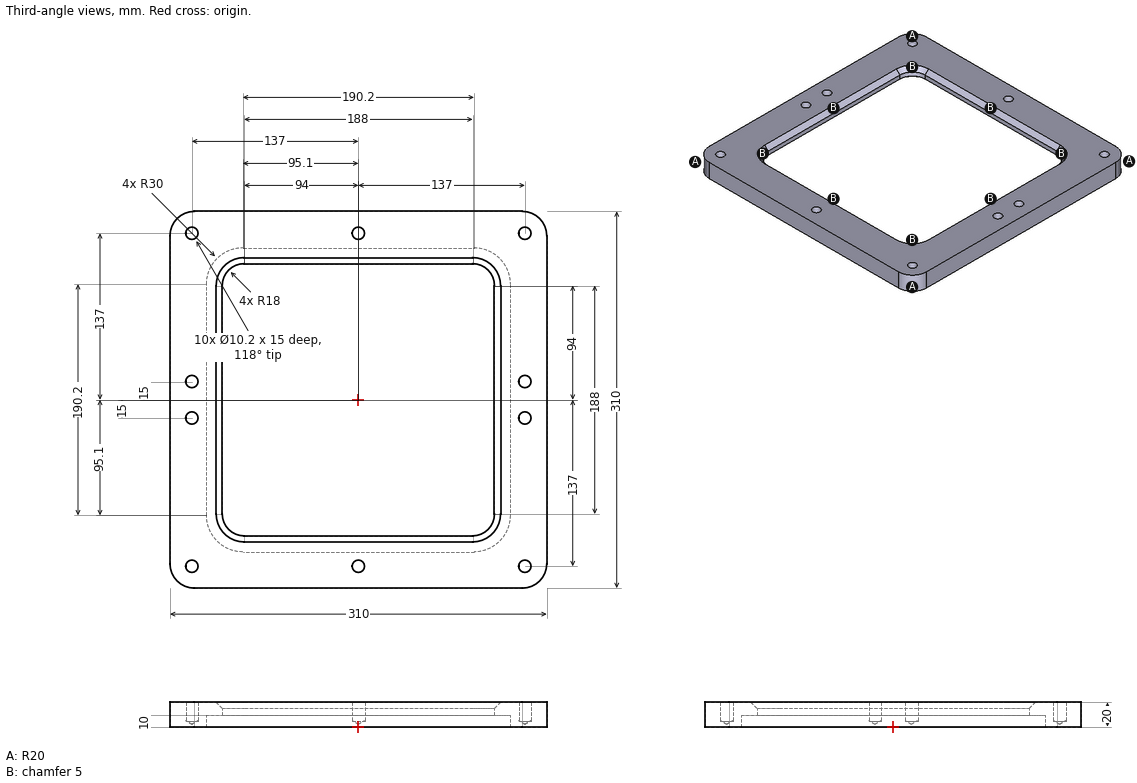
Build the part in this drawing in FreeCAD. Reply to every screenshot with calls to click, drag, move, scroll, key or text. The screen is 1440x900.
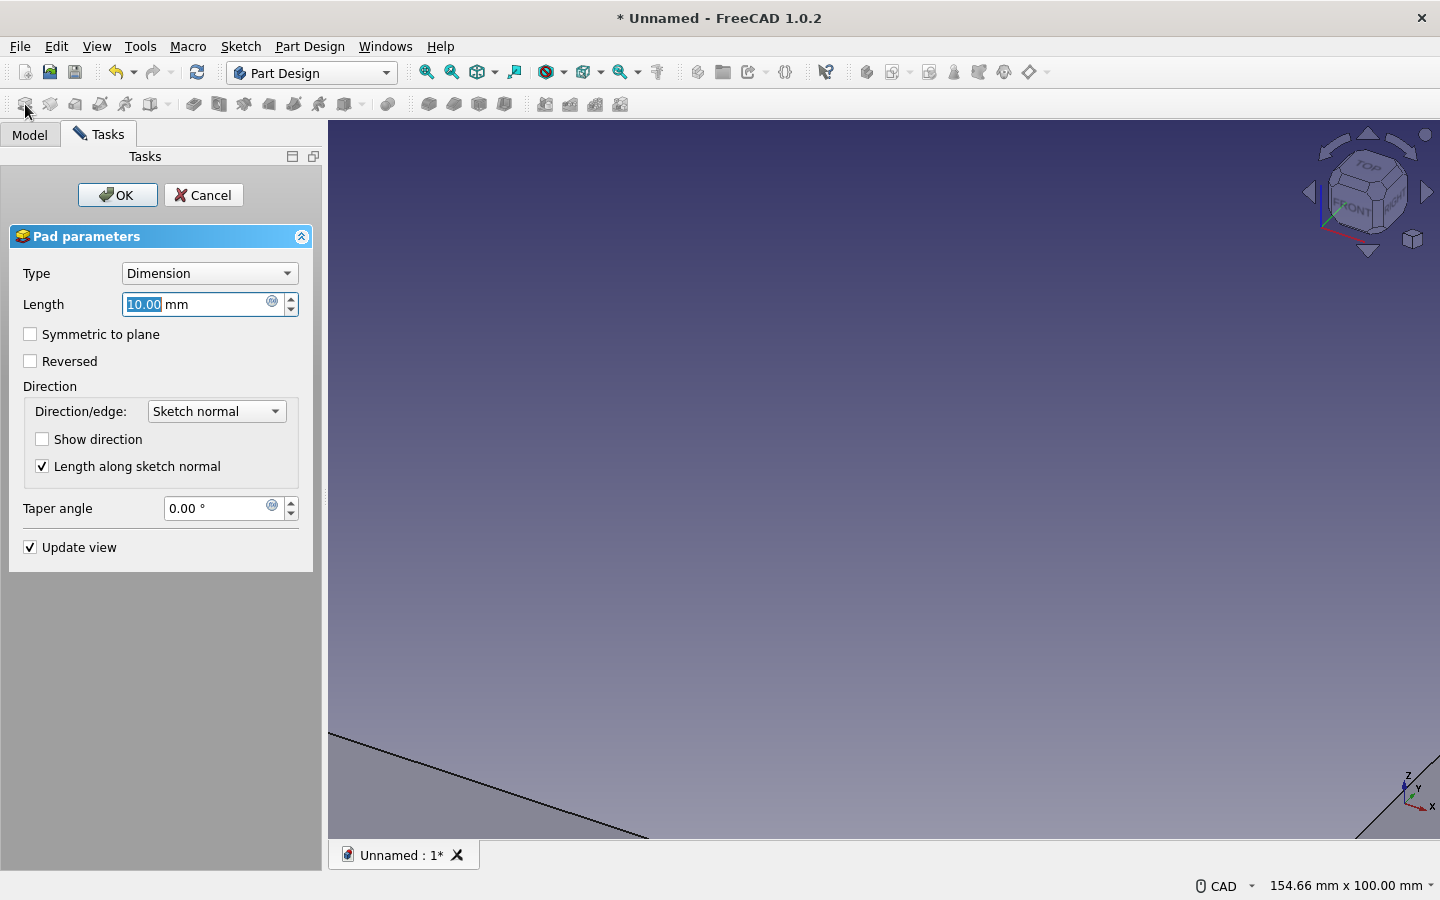
text(20)
key(Tab)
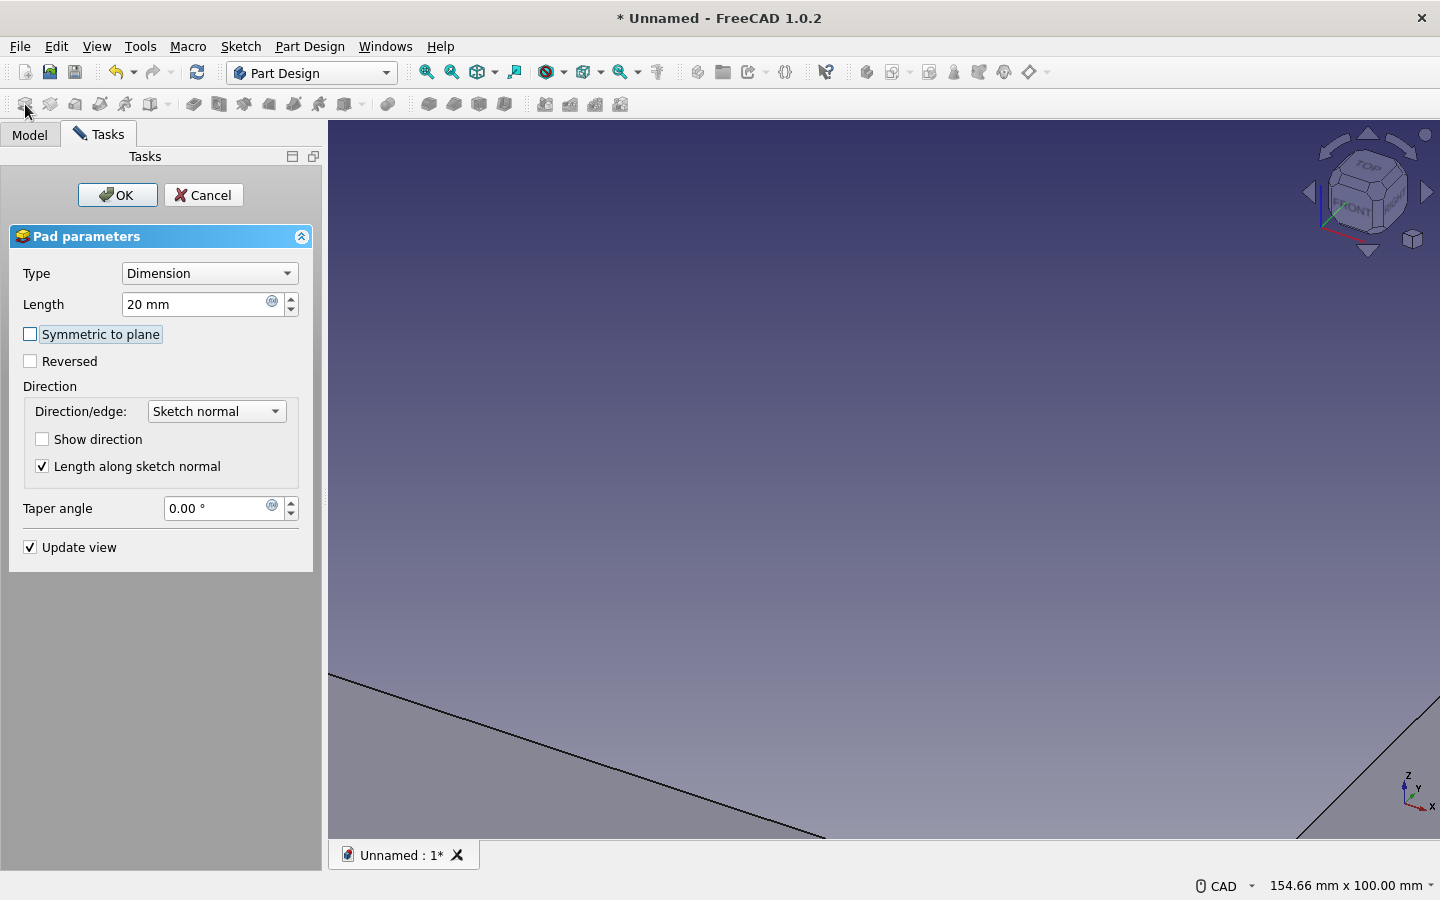
click(118, 195)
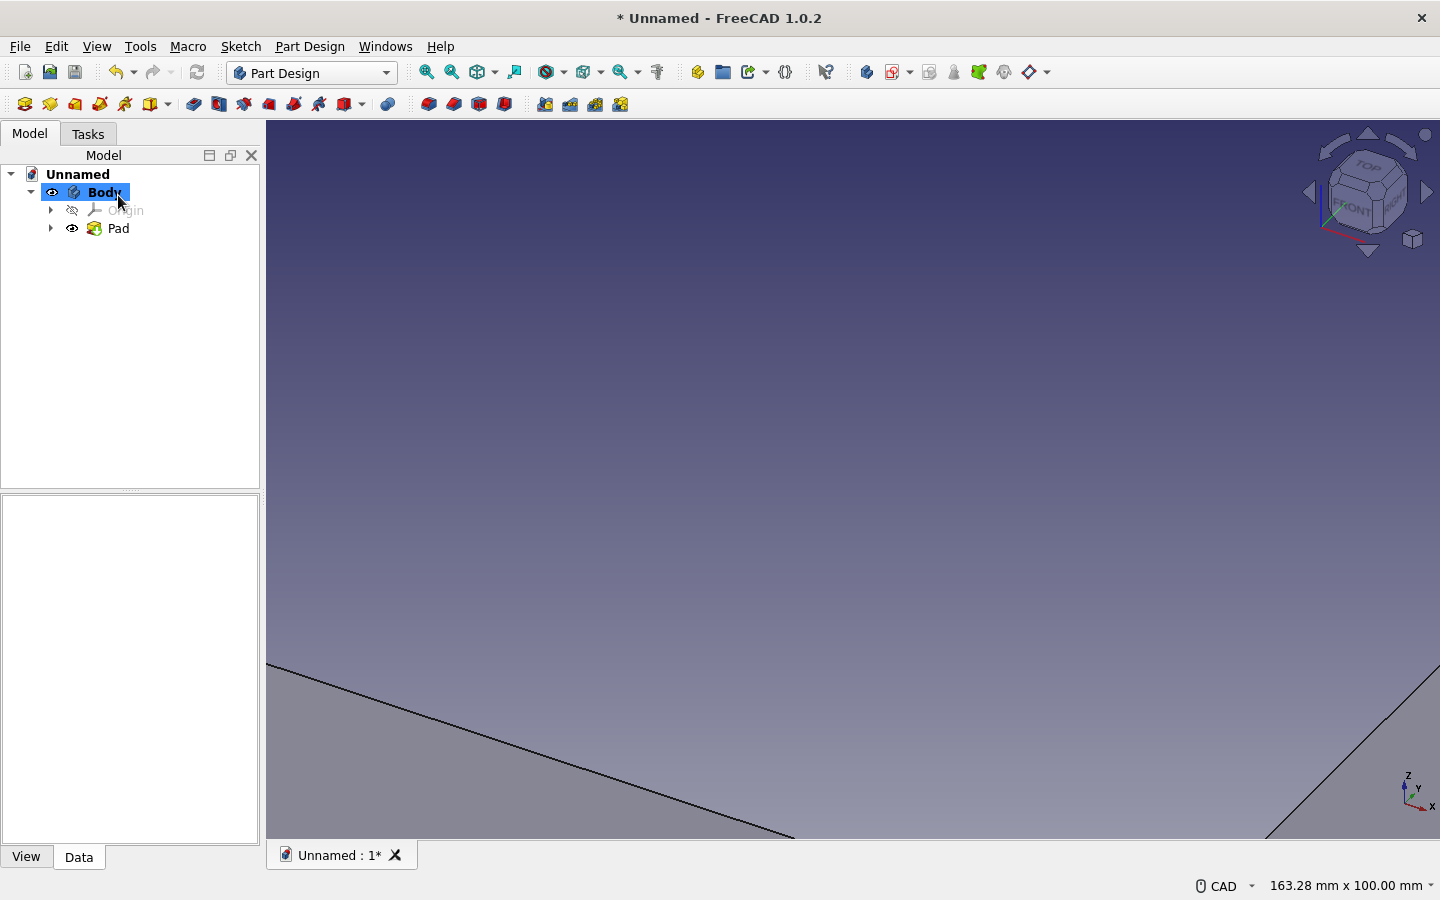
click(427, 72)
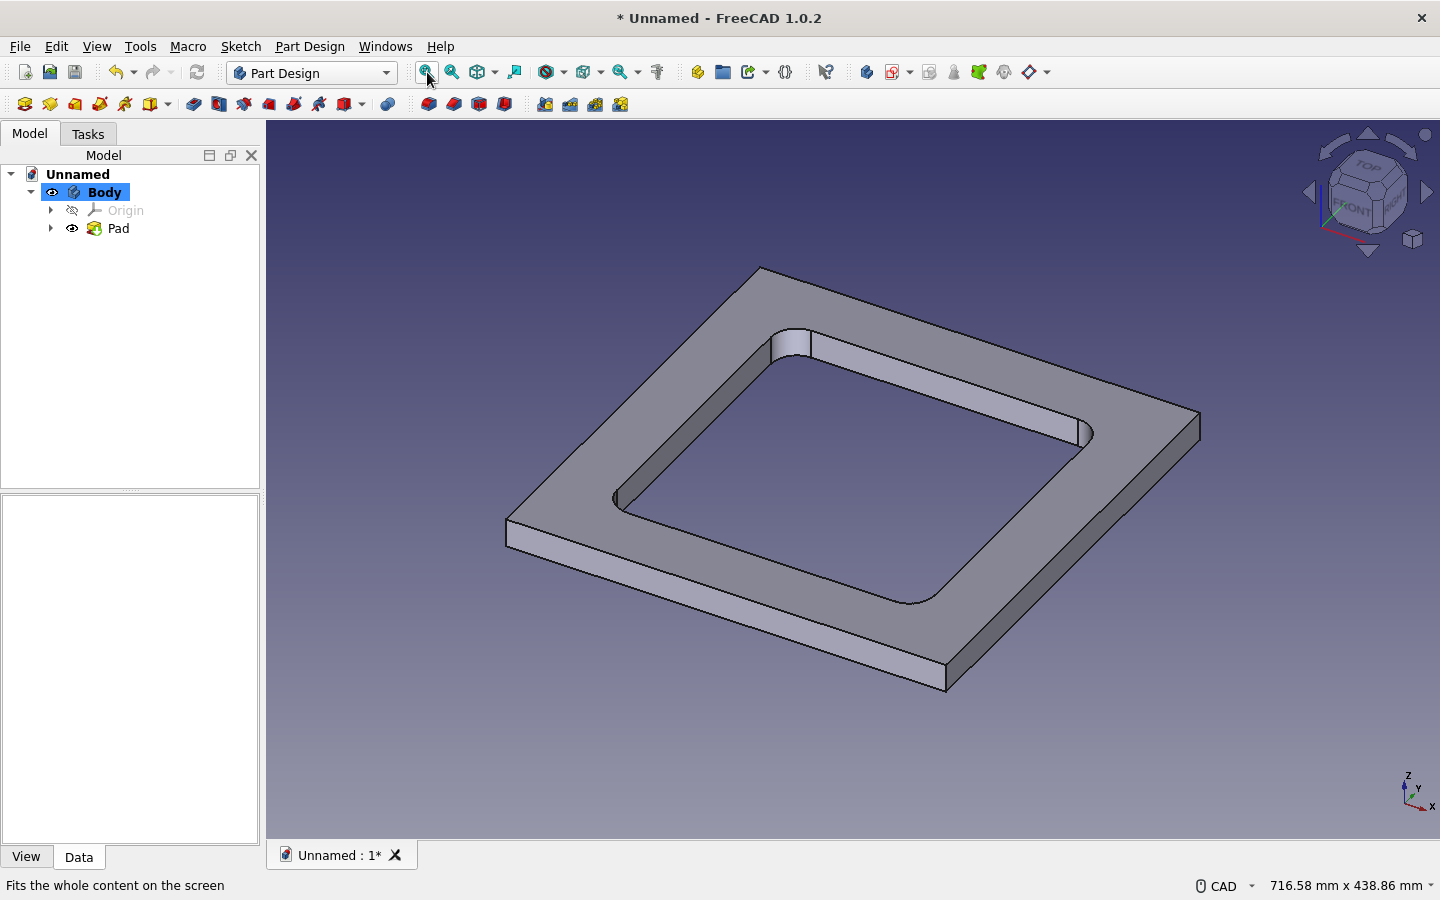
click(946, 677)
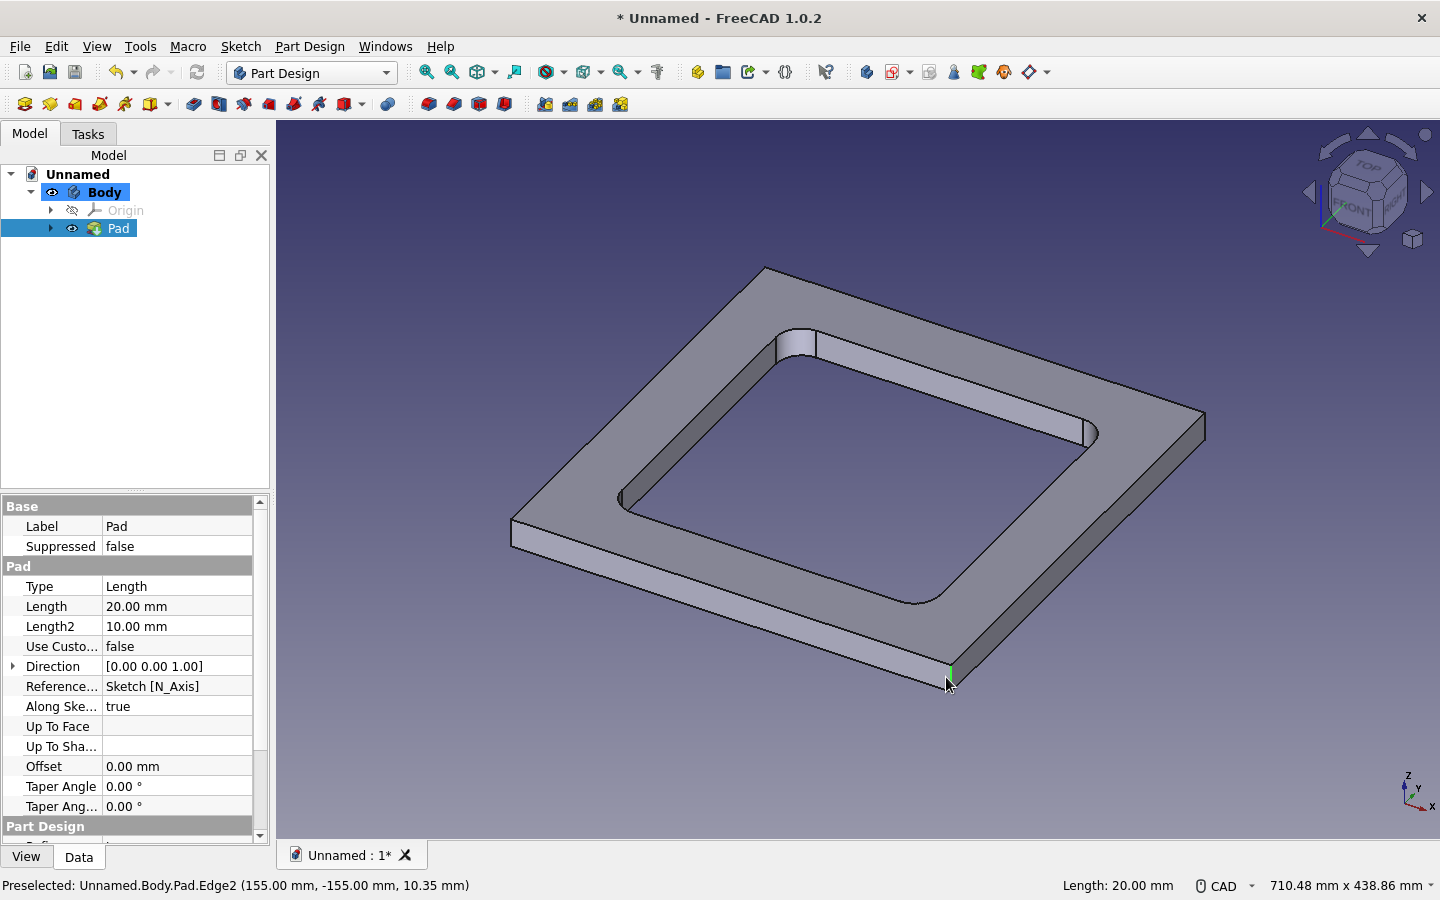
key(0)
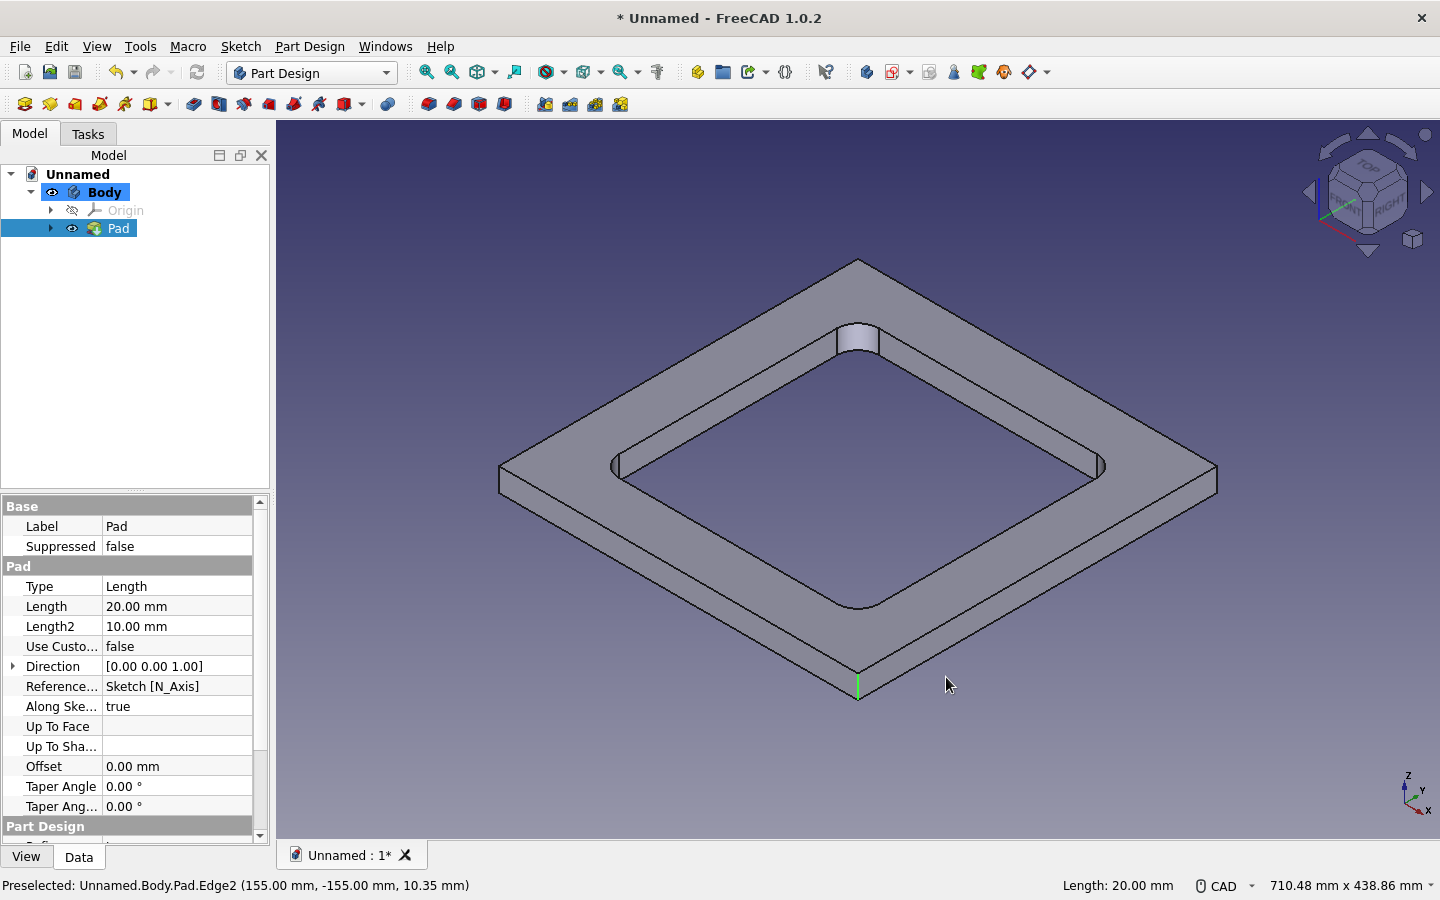
key(2)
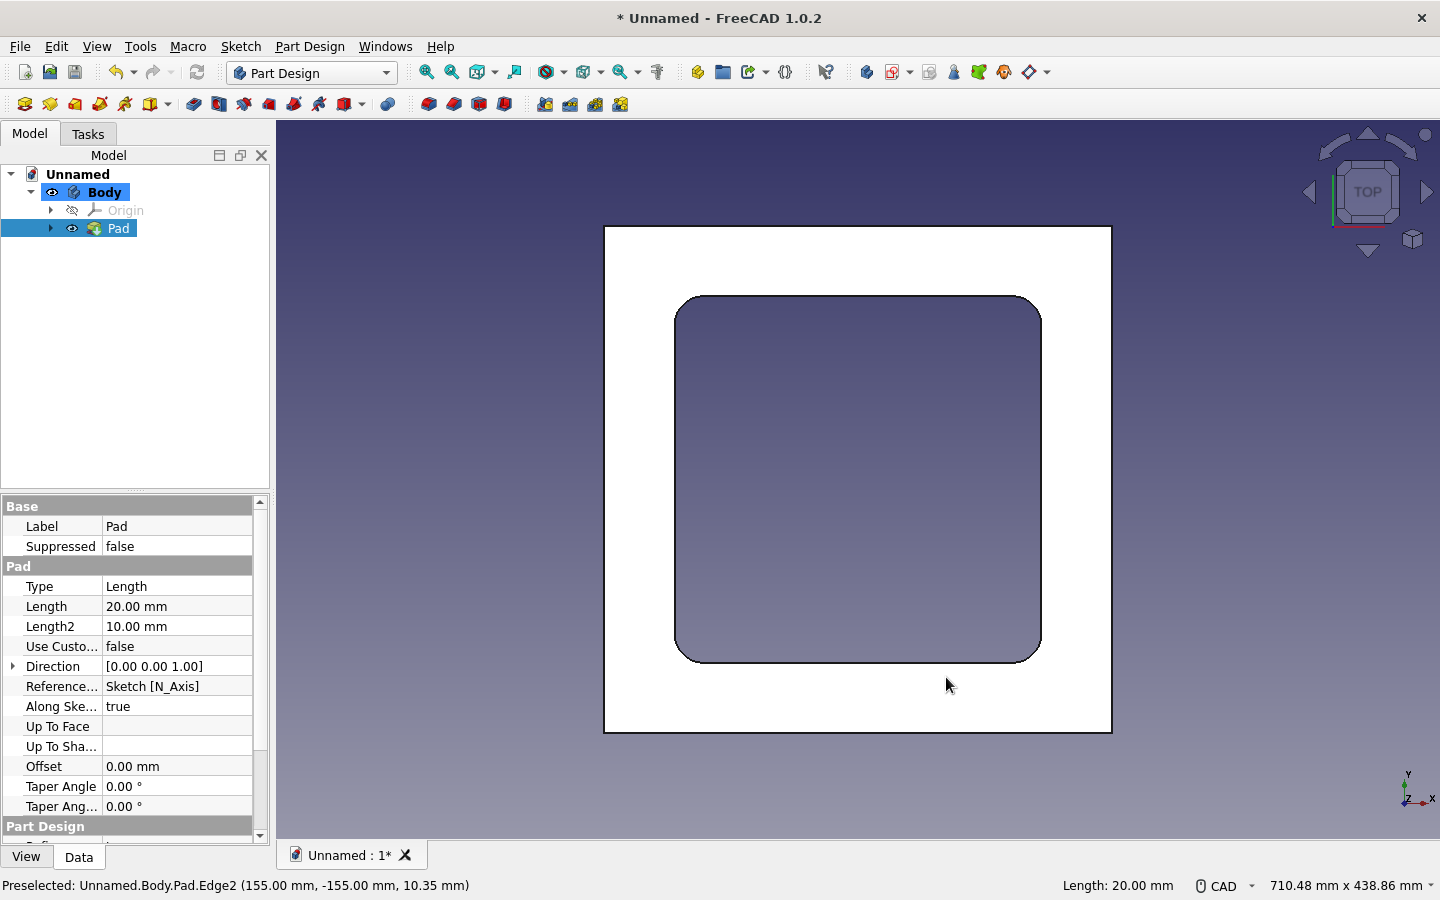
key(1)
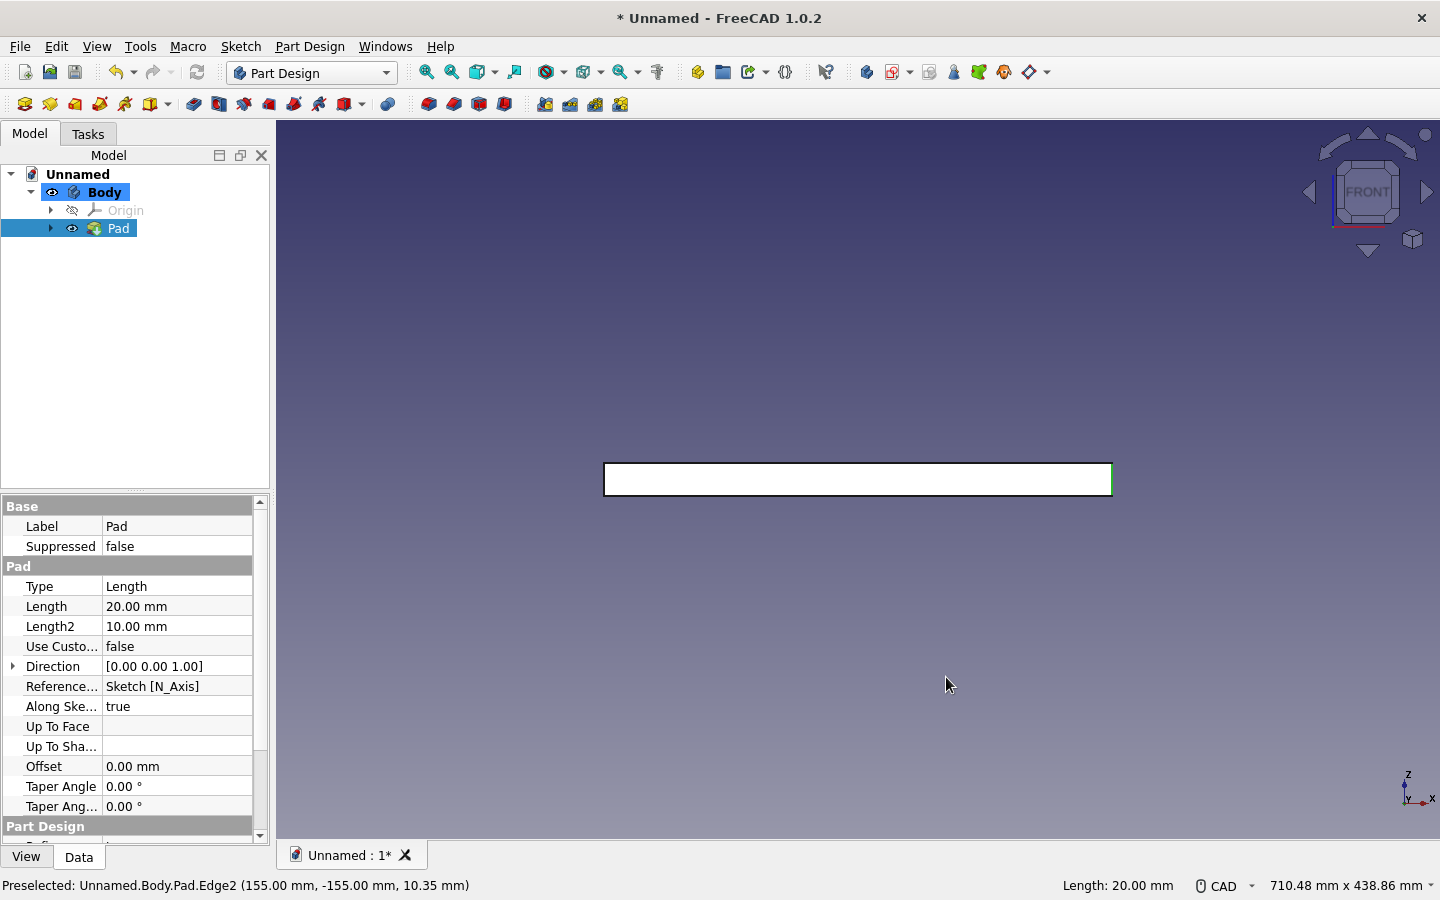
click(427, 72)